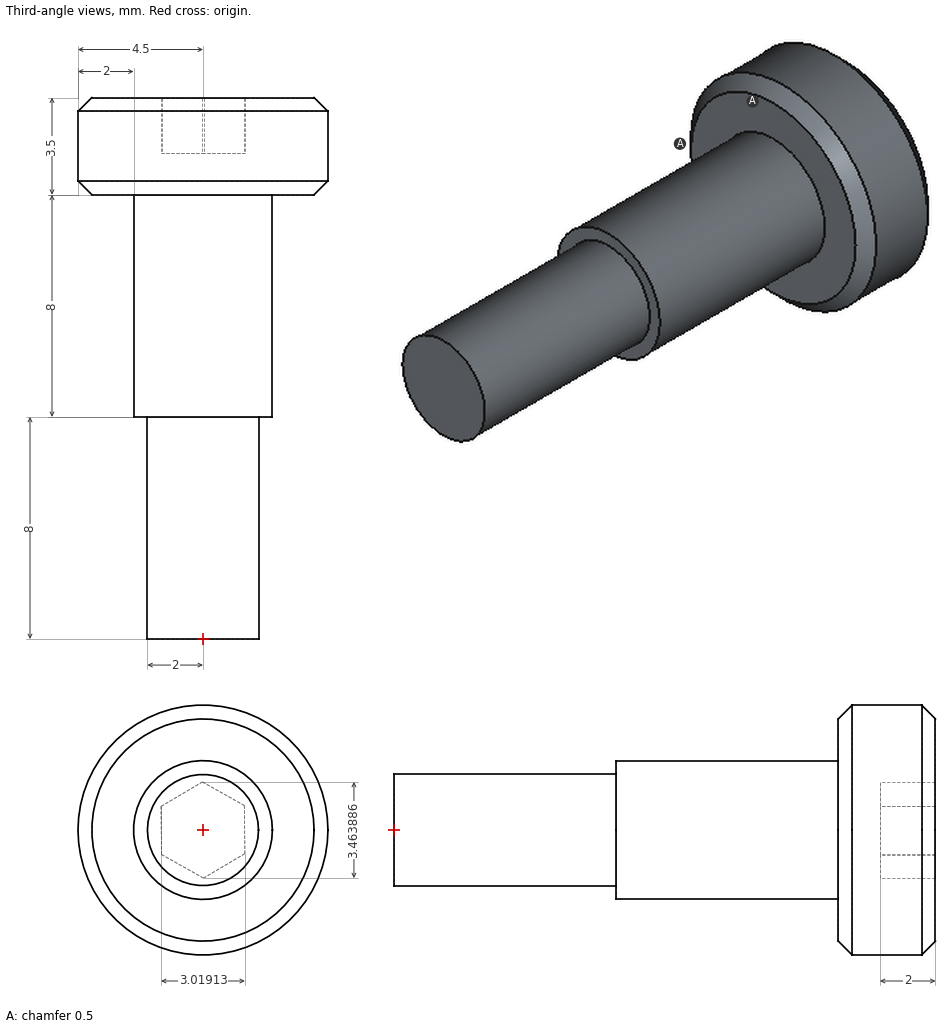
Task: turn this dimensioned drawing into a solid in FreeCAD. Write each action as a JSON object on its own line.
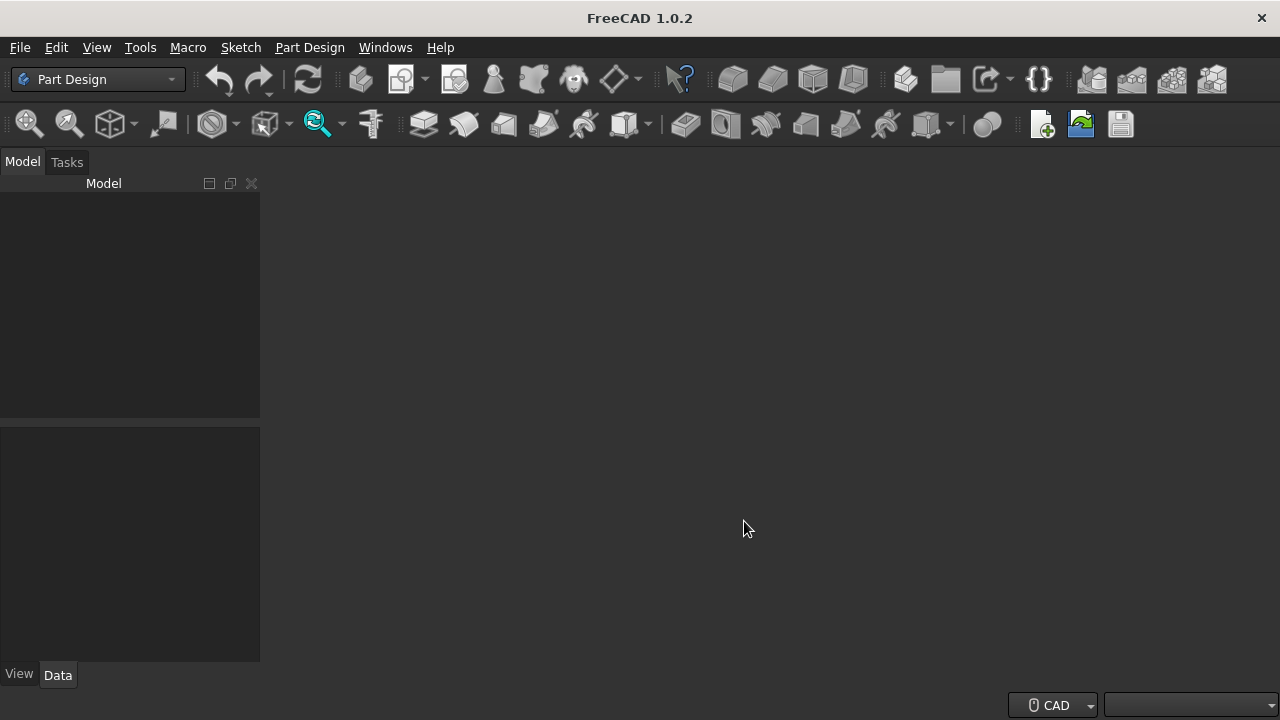
{"action": "left_click", "coordinate": [1042, 124]}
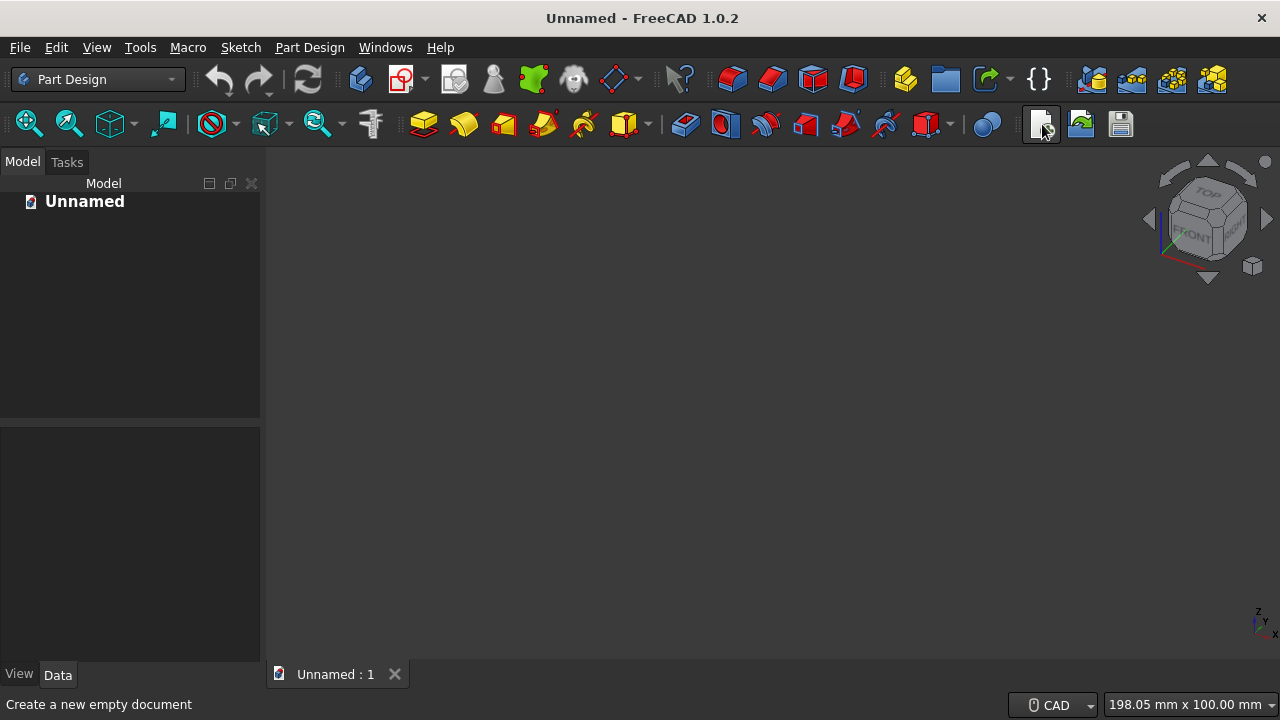
{"action": "left_click", "coordinate": [402, 80]}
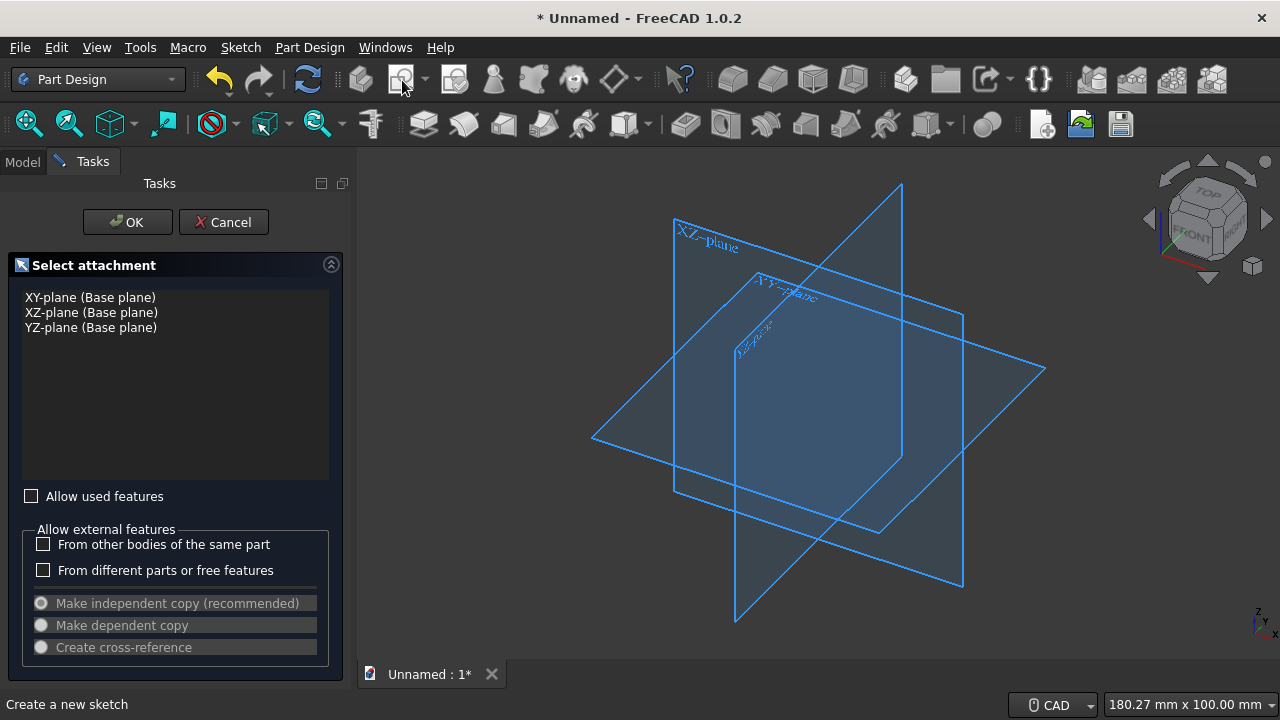
{"action": "left_click", "coordinate": [82, 298]}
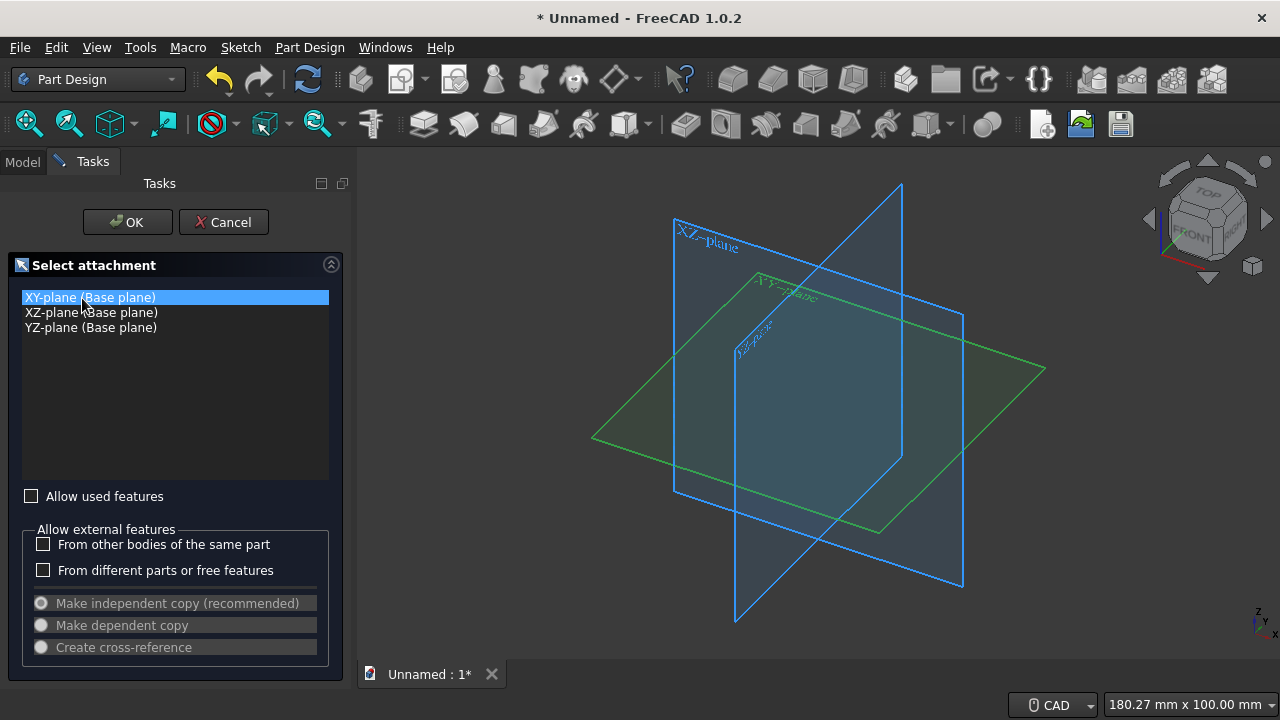
{"action": "left_click", "coordinate": [128, 222]}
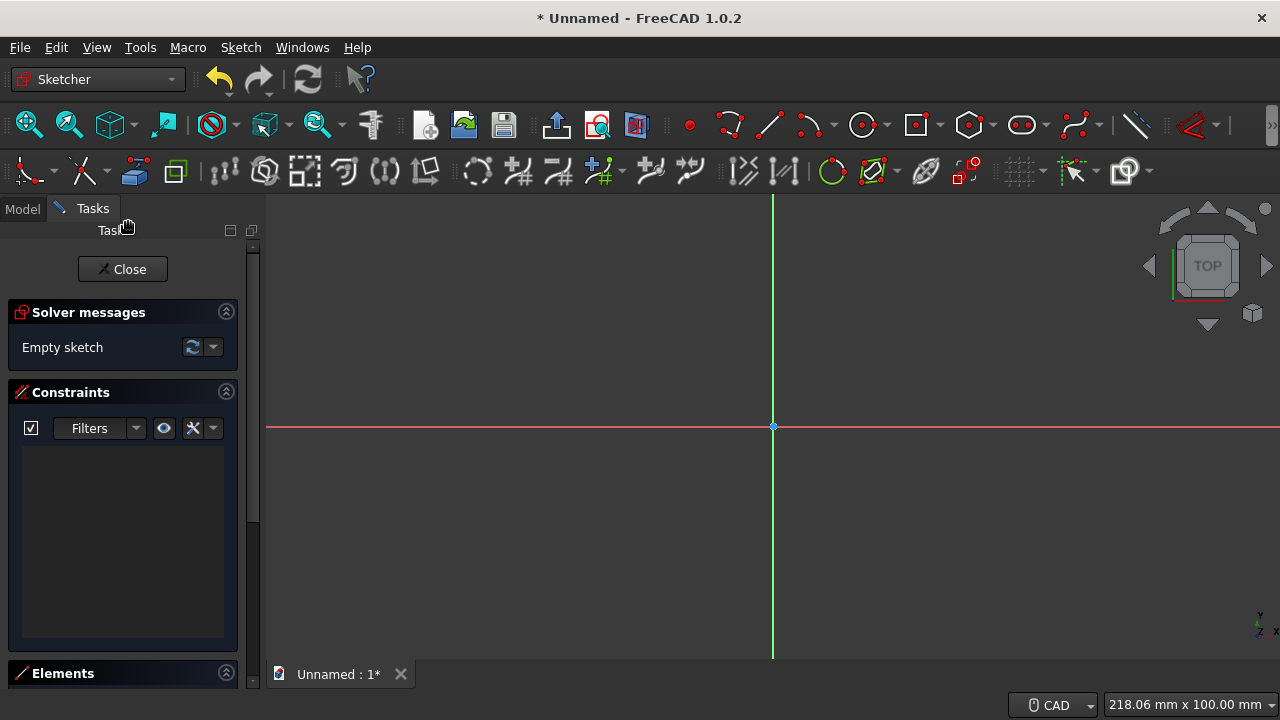
{"action": "scroll", "coordinate": [788, 362], "scroll_direction": "up", "scroll_amount": 6}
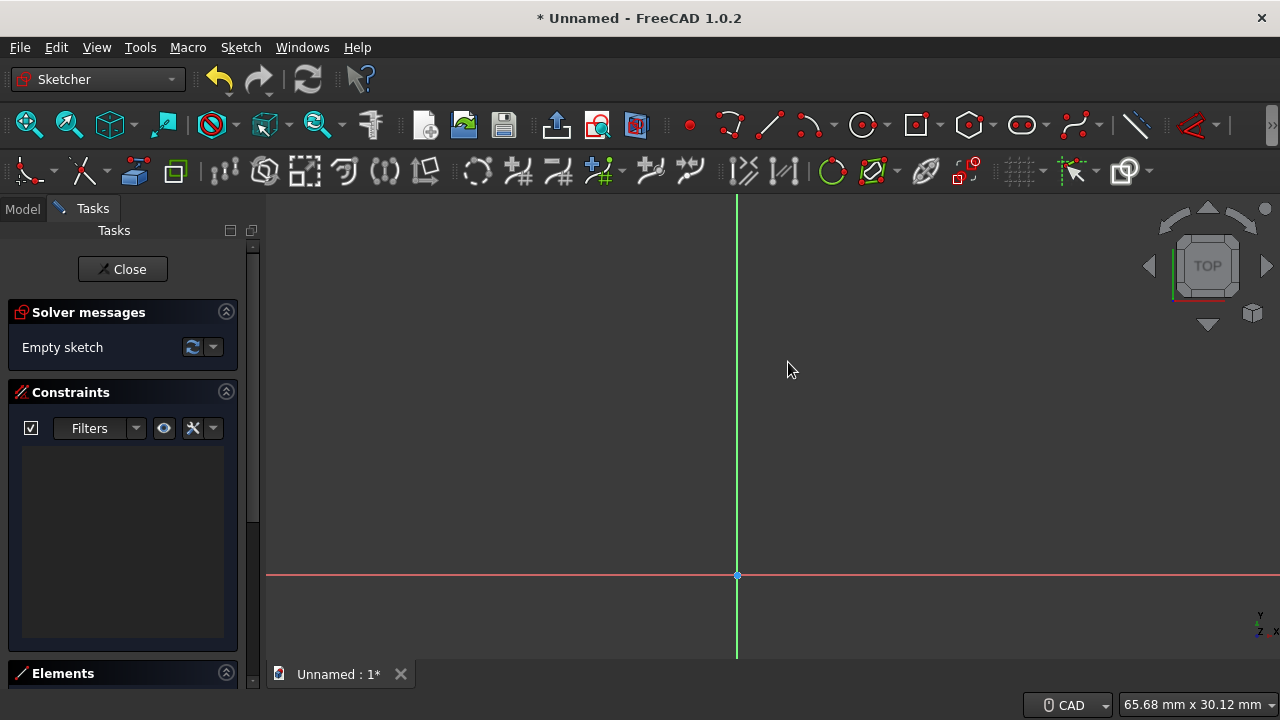
{"action": "key", "text": "g m"}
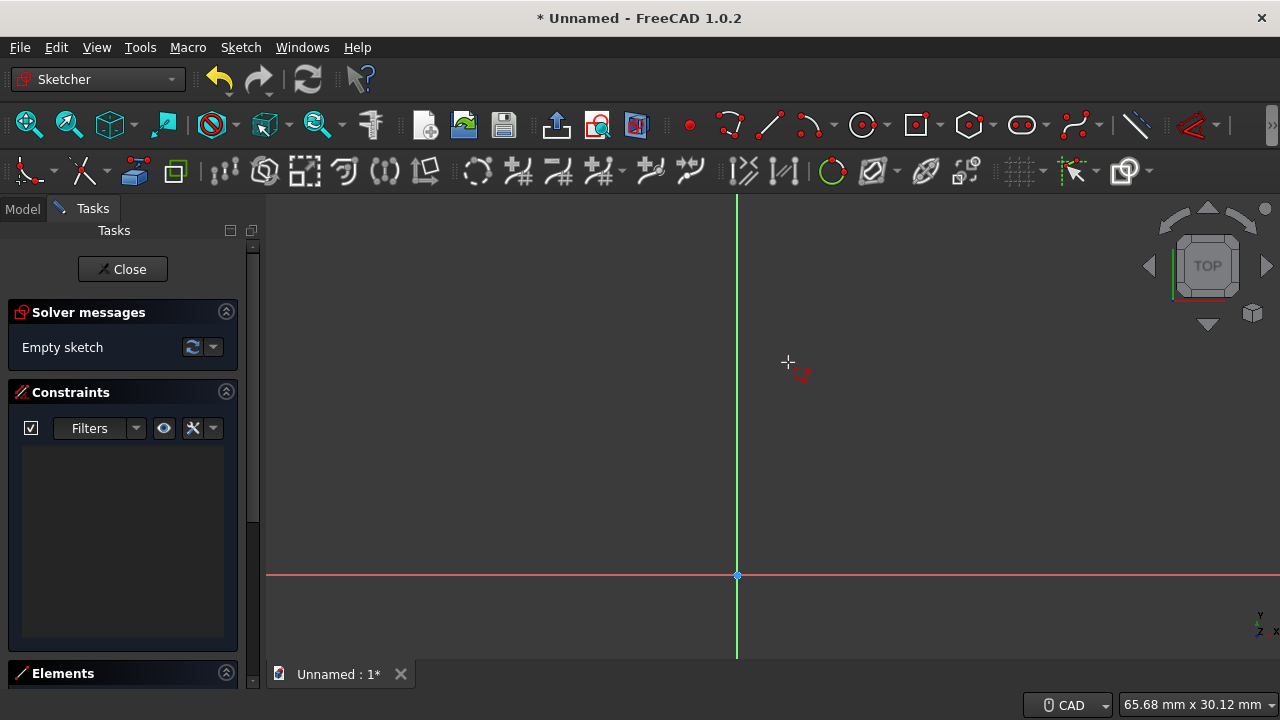
{"action": "left_click", "coordinate": [737, 575]}
{"action": "left_click", "coordinate": [728, 274]}
{"action": "left_click", "coordinate": [668, 274]}
{"action": "left_click", "coordinate": [668, 328]}
{"action": "left_click", "coordinate": [698, 328]}
{"action": "left_click", "coordinate": [698, 452]}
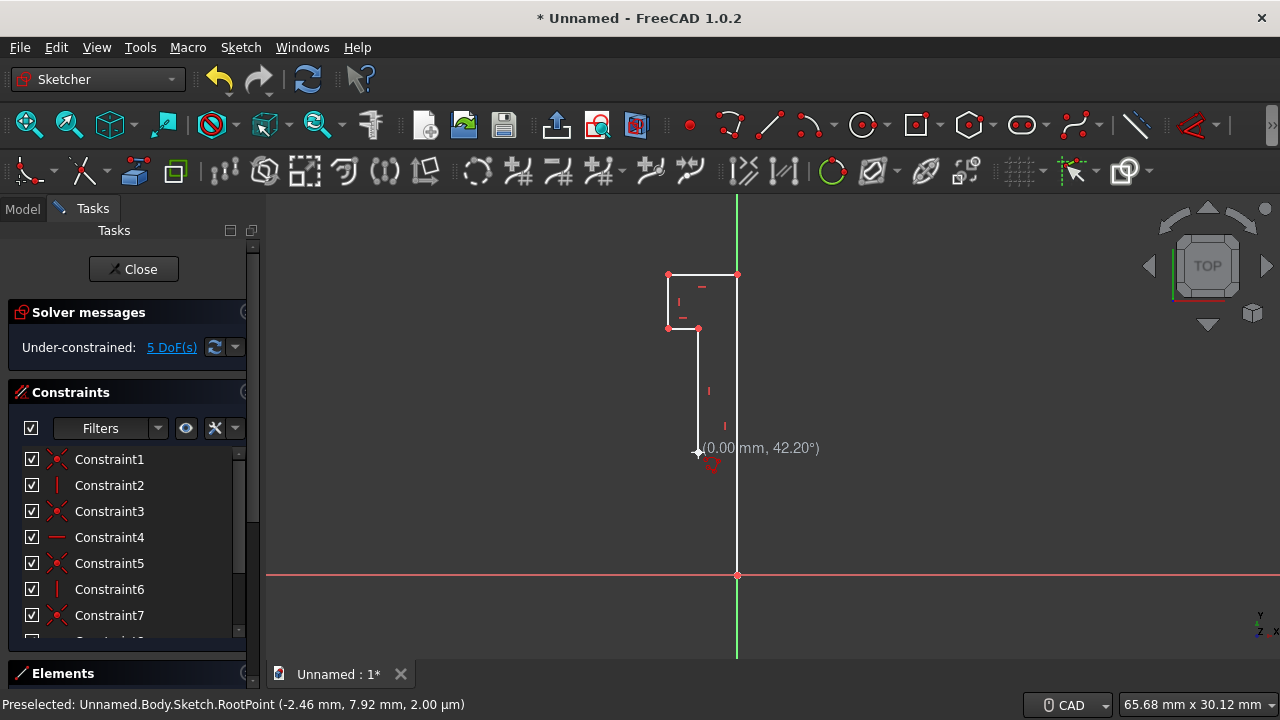
{"action": "scroll", "coordinate": [706, 452], "scroll_direction": "up", "scroll_amount": 4}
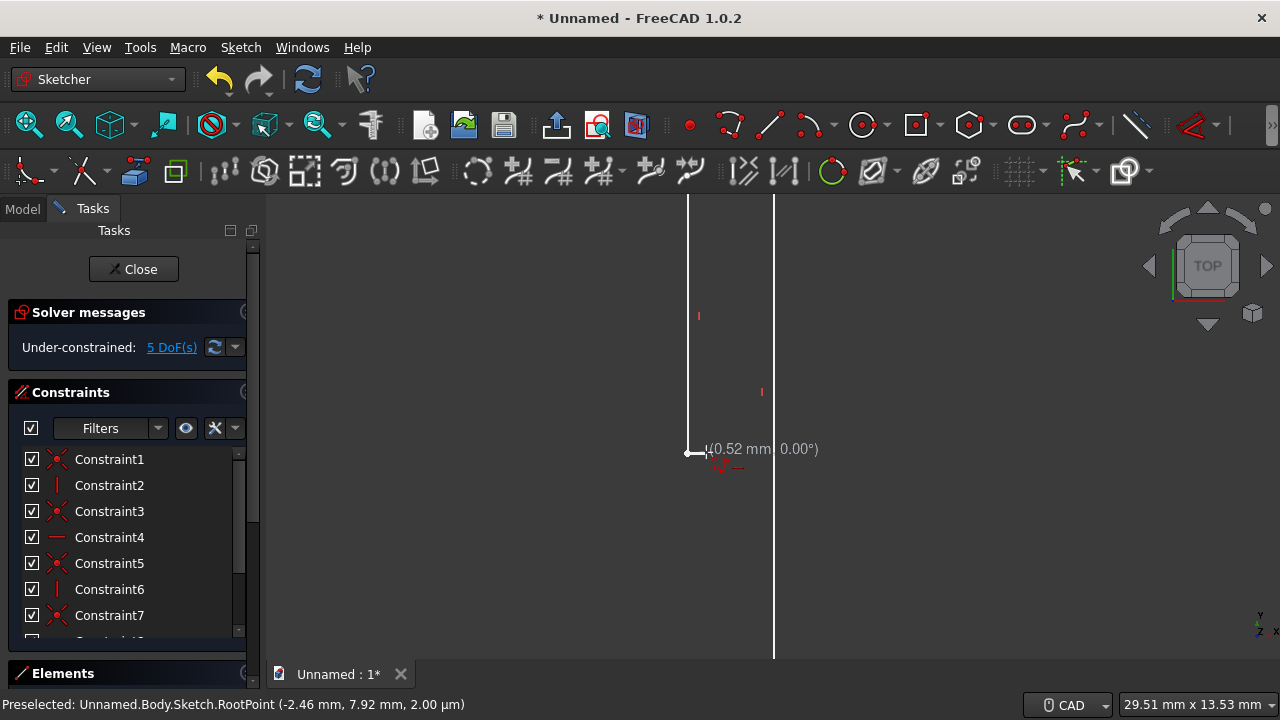
{"action": "left_click", "coordinate": [706, 451]}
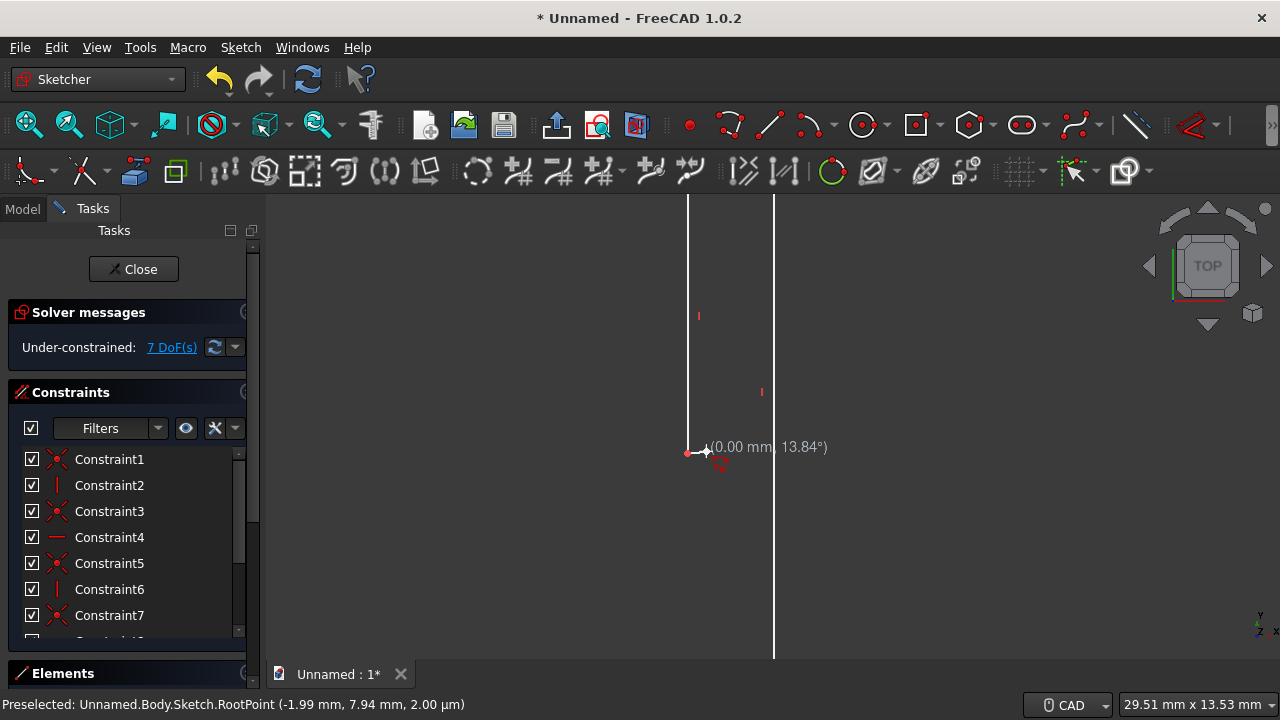
{"action": "scroll", "coordinate": [710, 456], "scroll_direction": "down", "scroll_amount": 4}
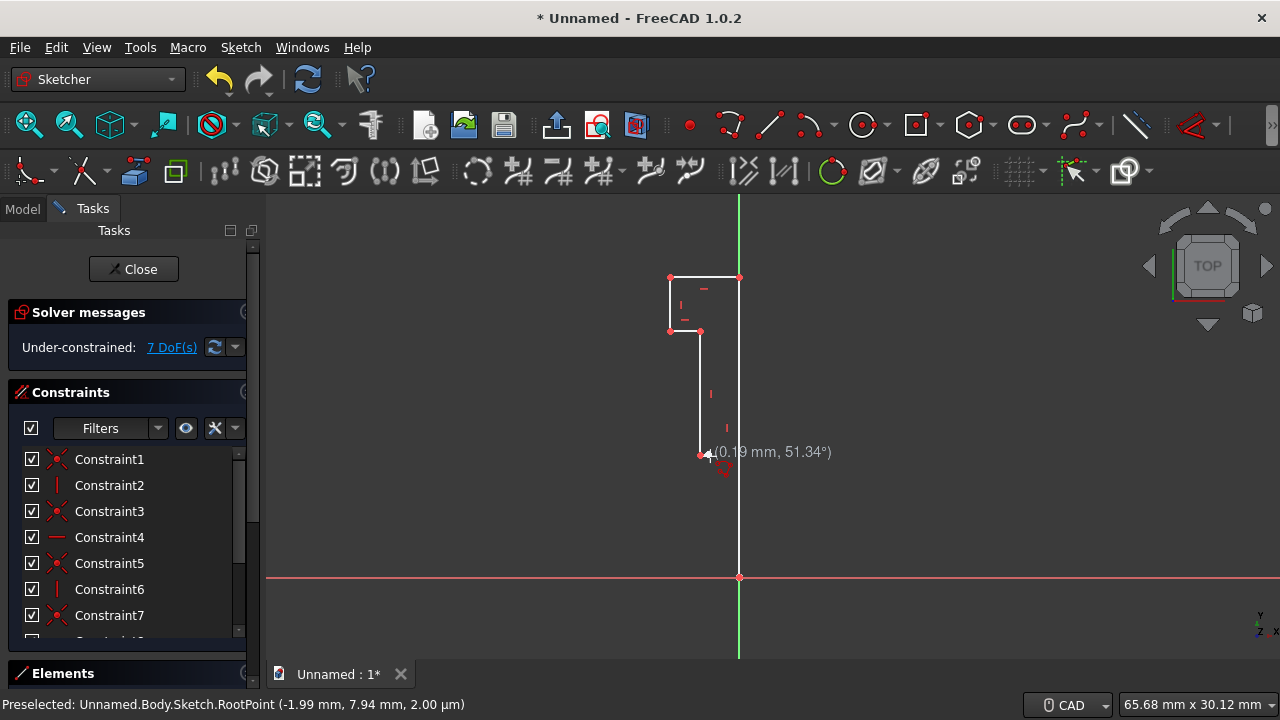
{"action": "left_click", "coordinate": [708, 569]}
{"action": "left_click", "coordinate": [739, 578]}
{"action": "key", "text": "Escape"}
{"action": "key", "text": "Escape"}